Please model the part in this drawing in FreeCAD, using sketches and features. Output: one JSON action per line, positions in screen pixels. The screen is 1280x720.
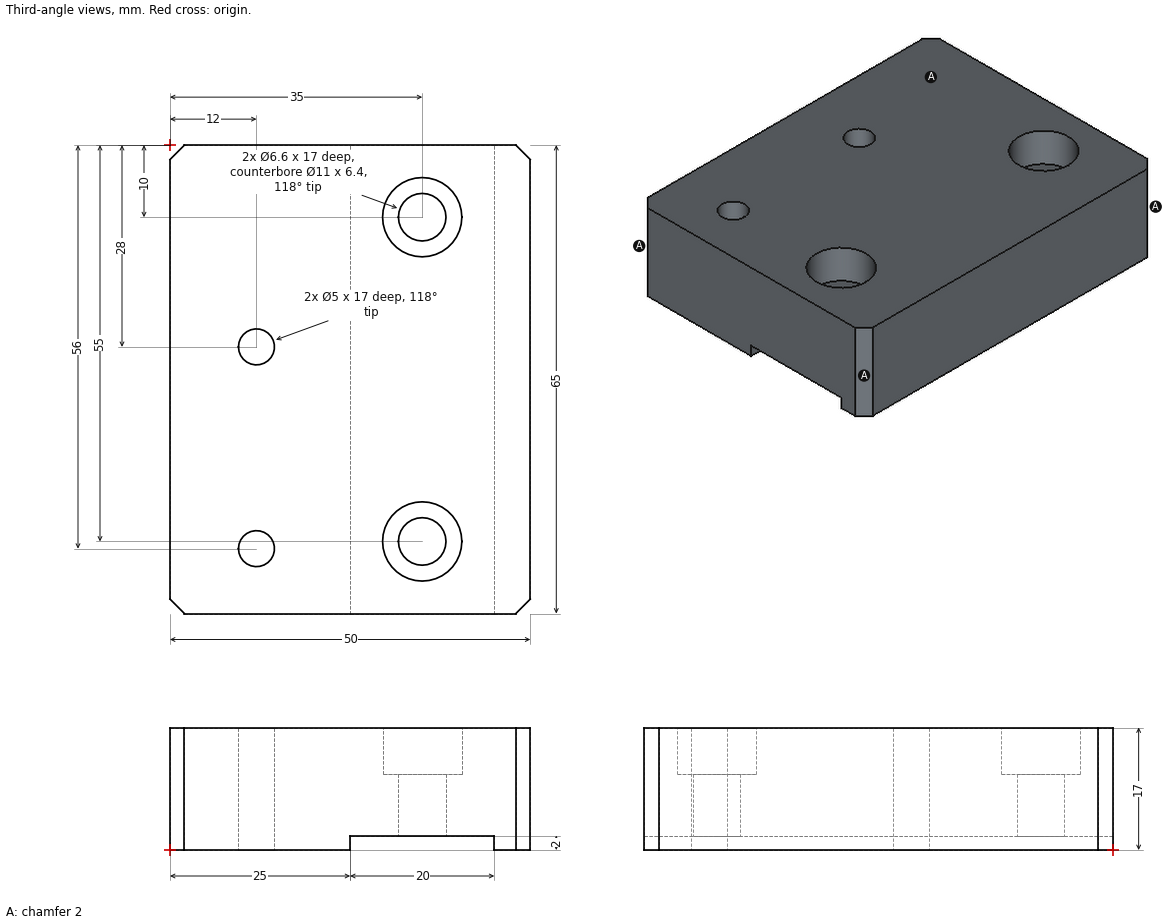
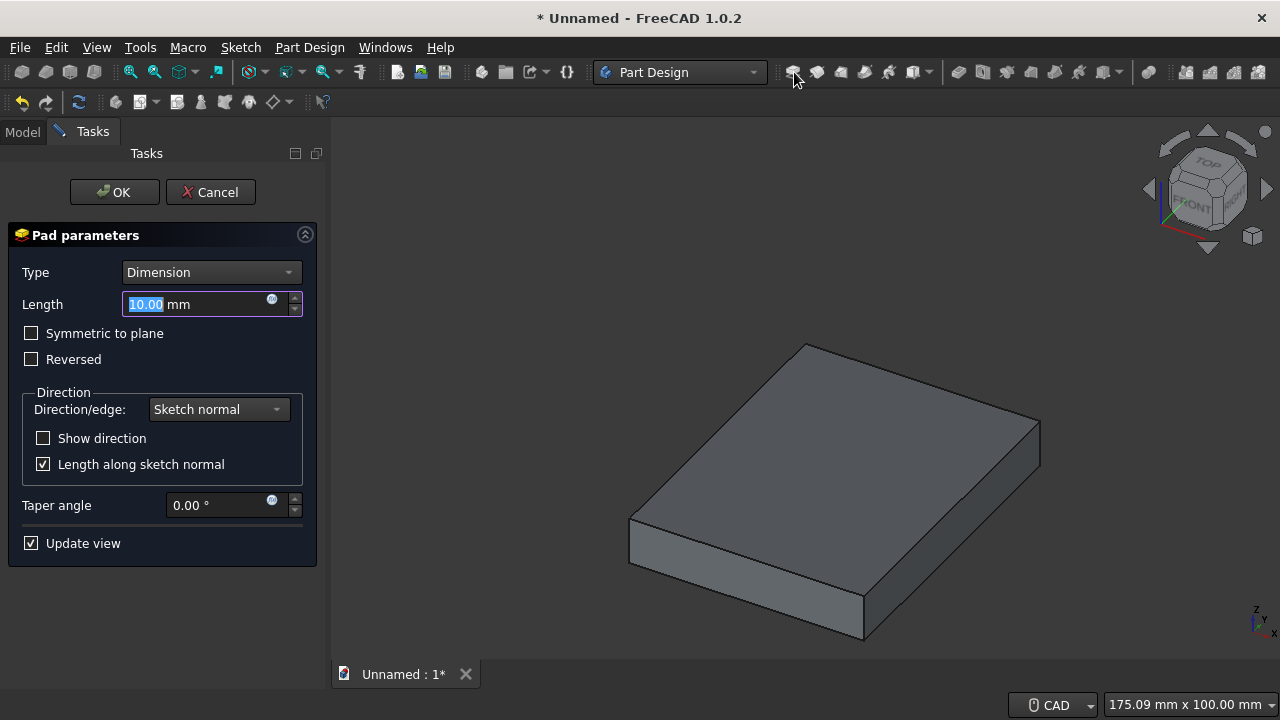
{"action": "type", "text": "17"}
{"action": "key", "text": "Tab"}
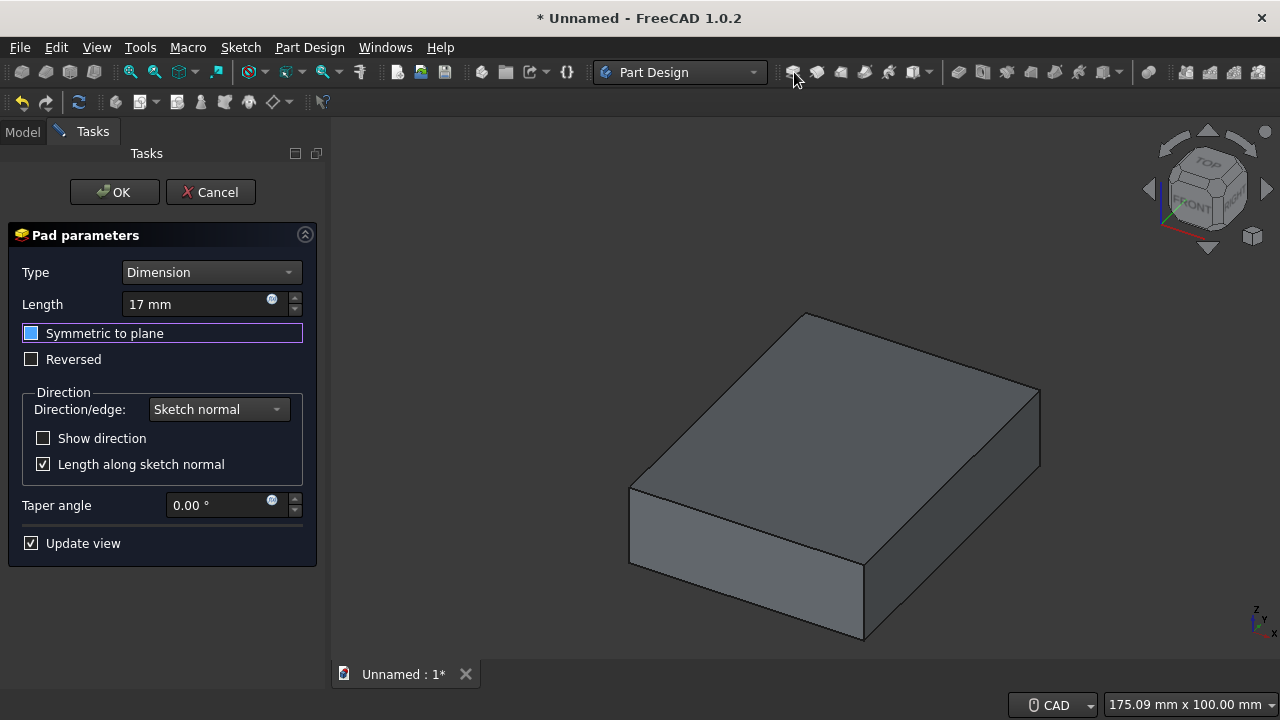
{"action": "left_click", "coordinate": [115, 192]}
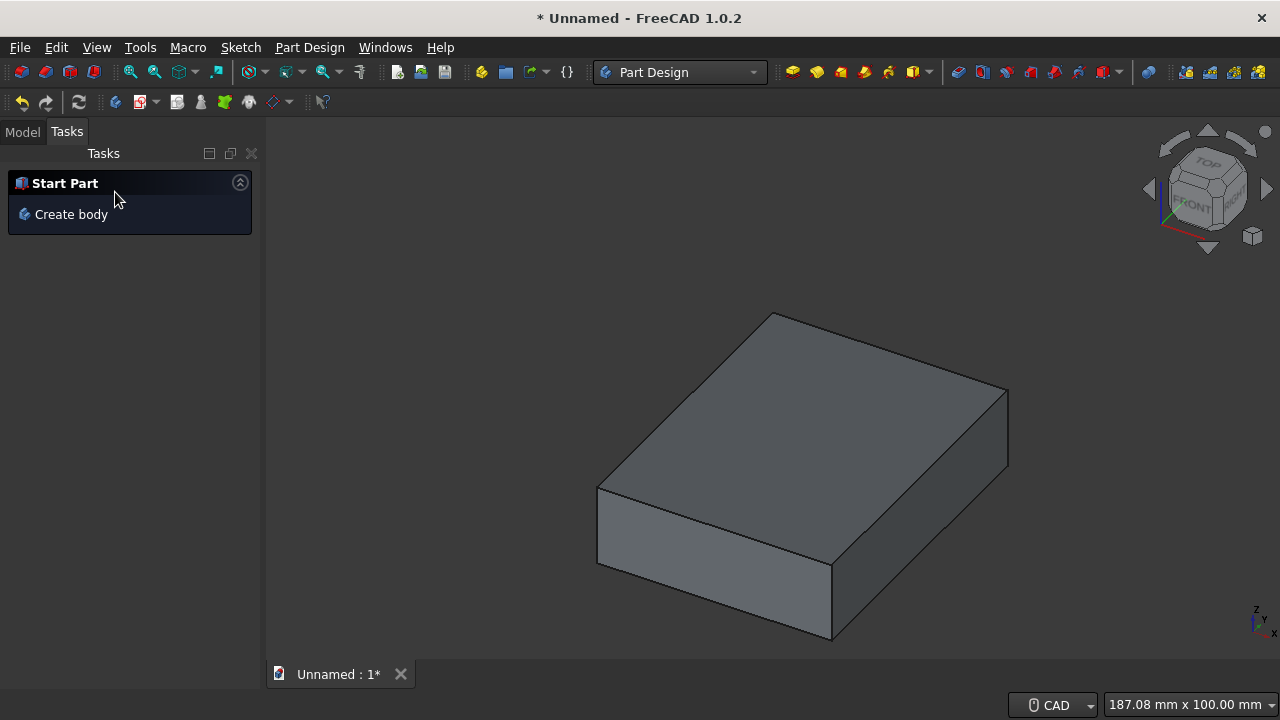
{"action": "left_click", "coordinate": [781, 585]}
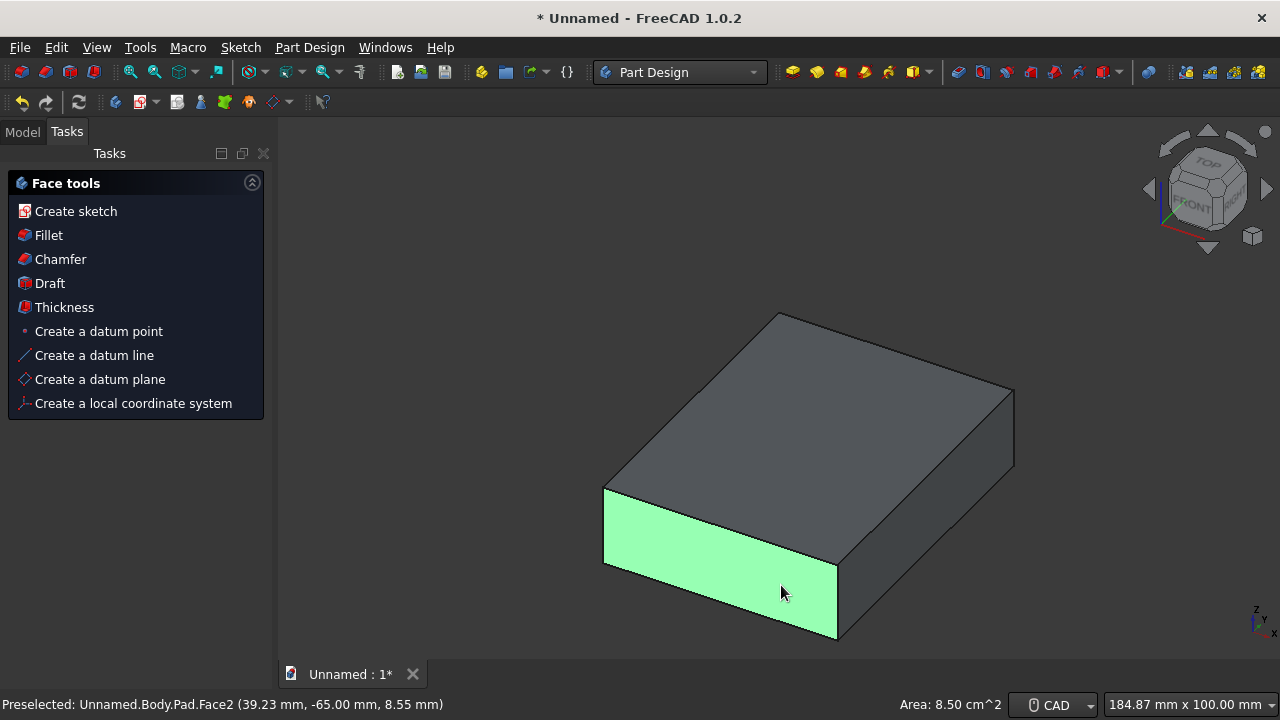
{"action": "left_click", "coordinate": [140, 102]}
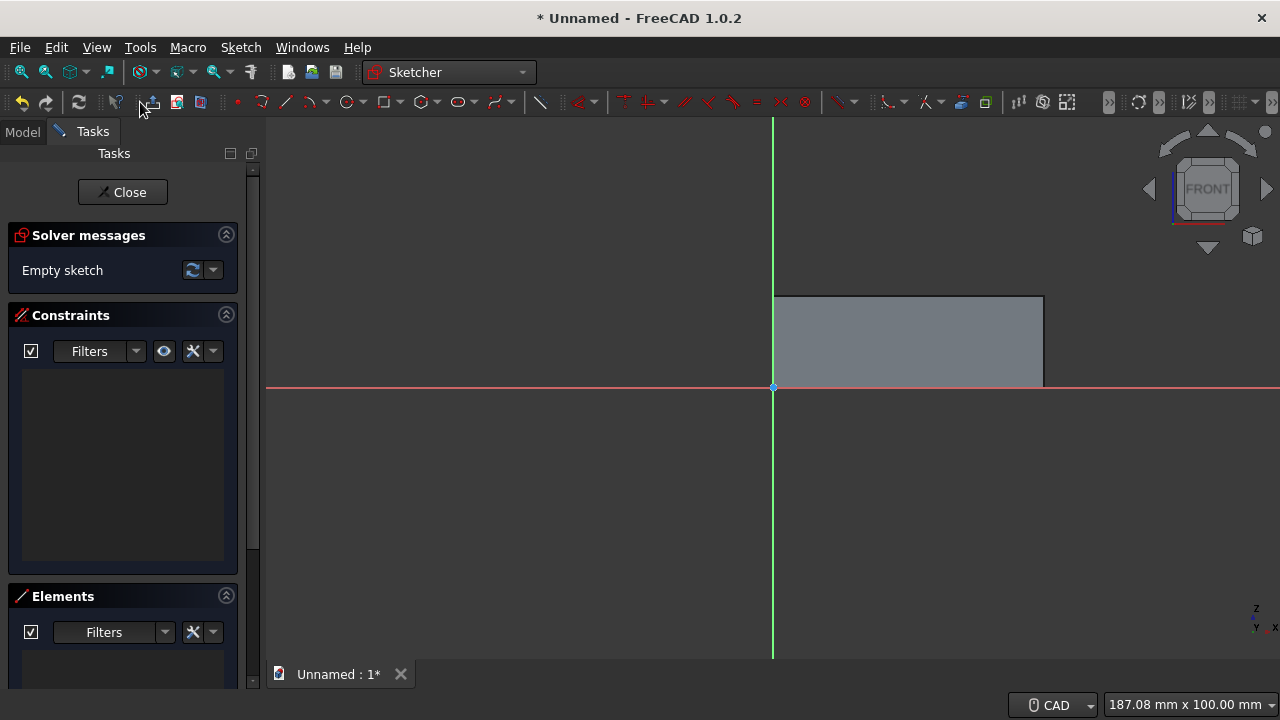
{"action": "scroll", "coordinate": [1050, 378], "scroll_direction": "up", "scroll_amount": 4}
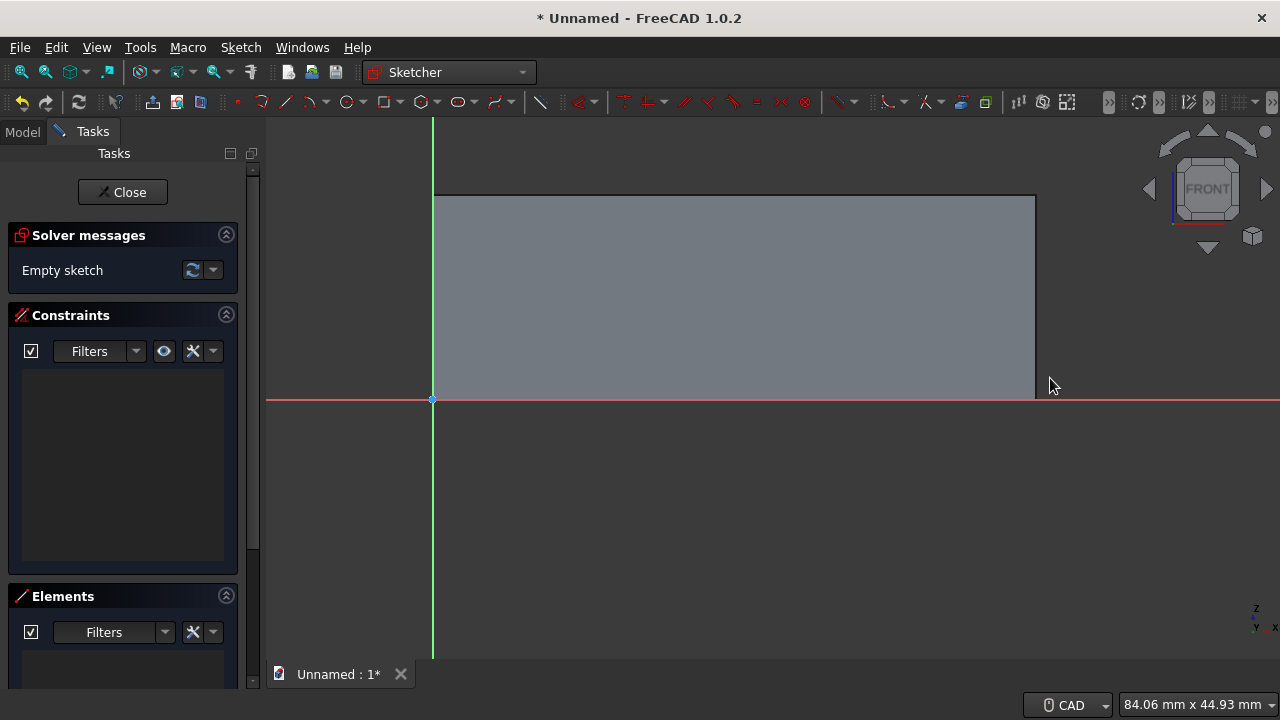
{"action": "left_click", "coordinate": [384, 102]}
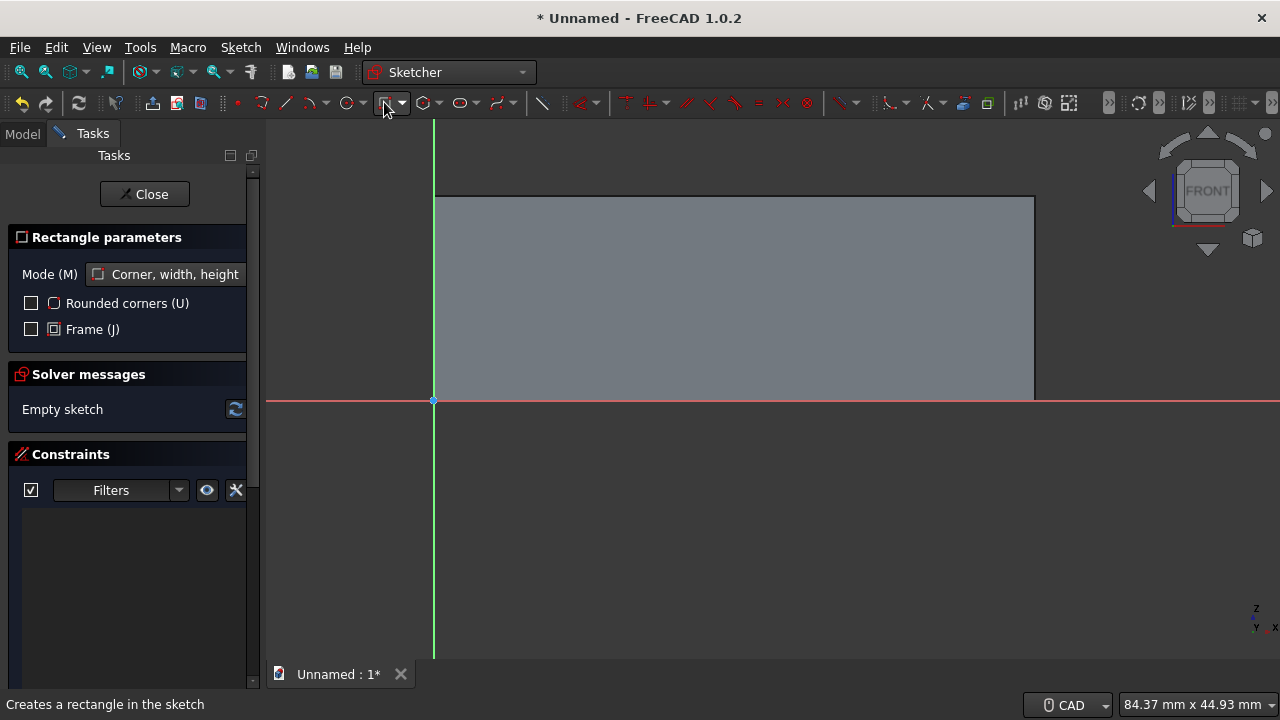
{"action": "left_click", "coordinate": [734, 377]}
{"action": "left_click", "coordinate": [975, 401]}
{"action": "key", "text": "Escape"}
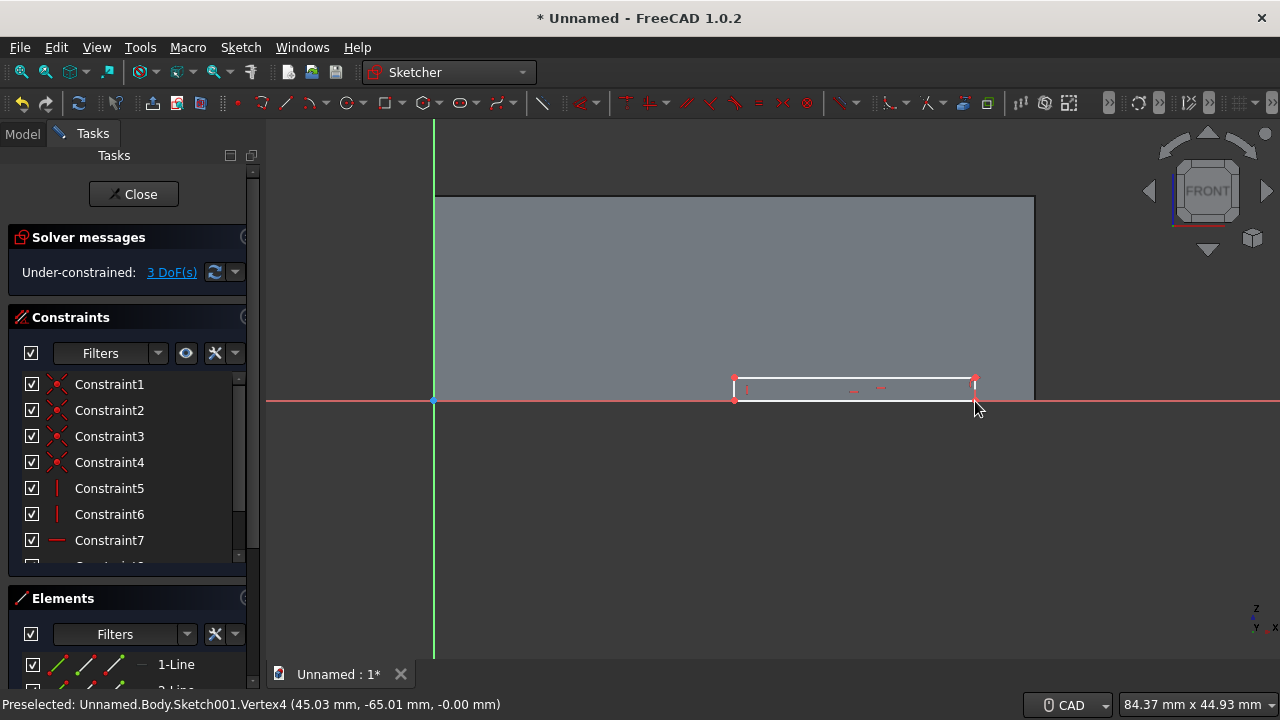
{"action": "scroll", "coordinate": [734, 387], "scroll_direction": "up", "scroll_amount": 3}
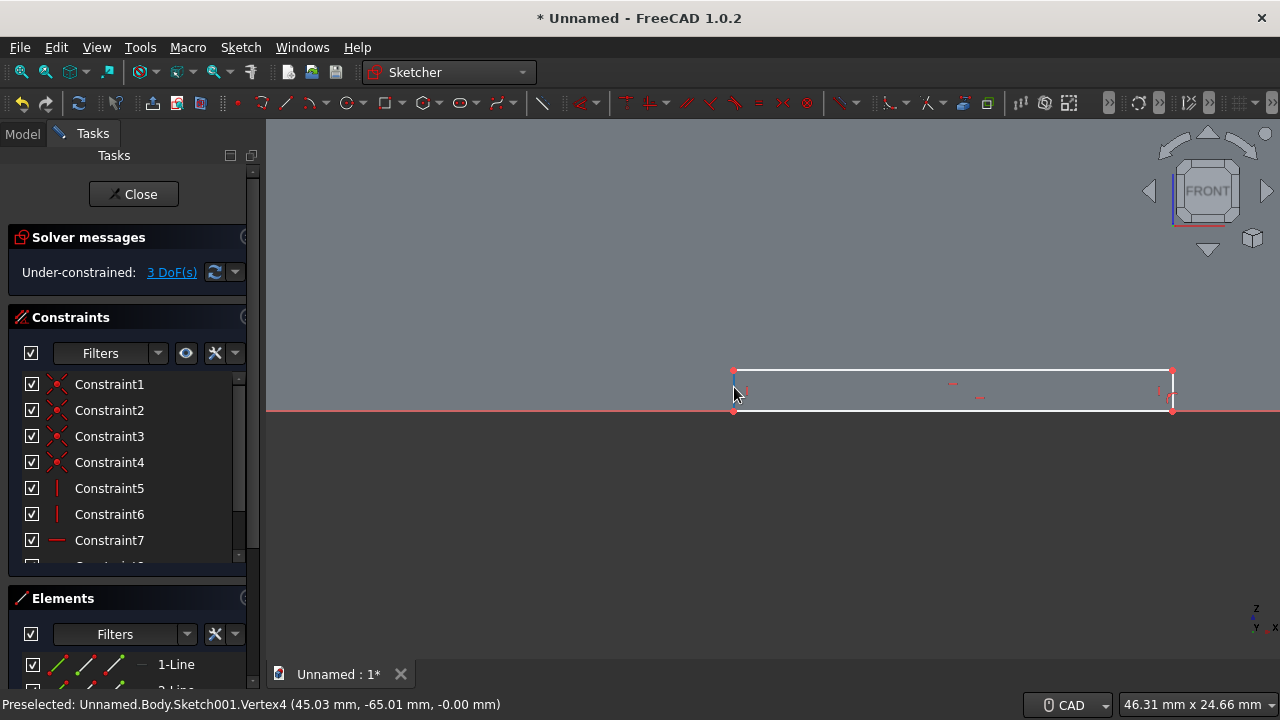
{"action": "left_click", "coordinate": [734, 387]}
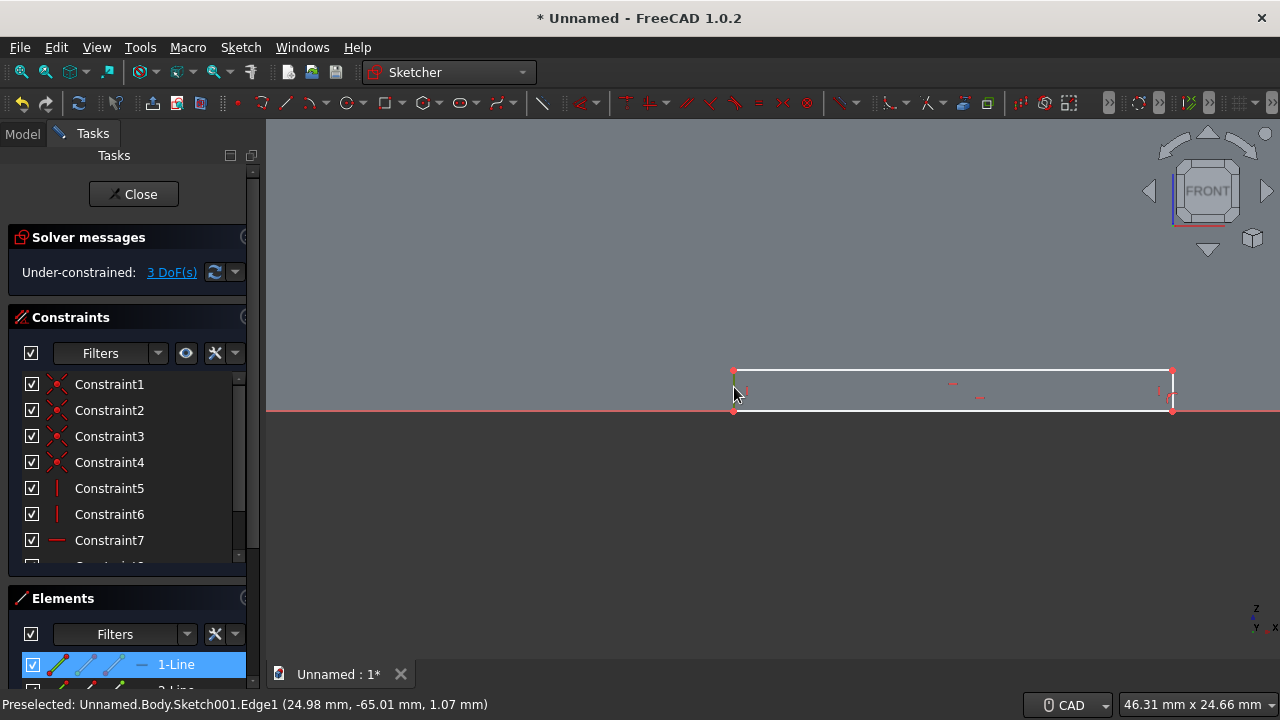
{"action": "key", "text": "i"}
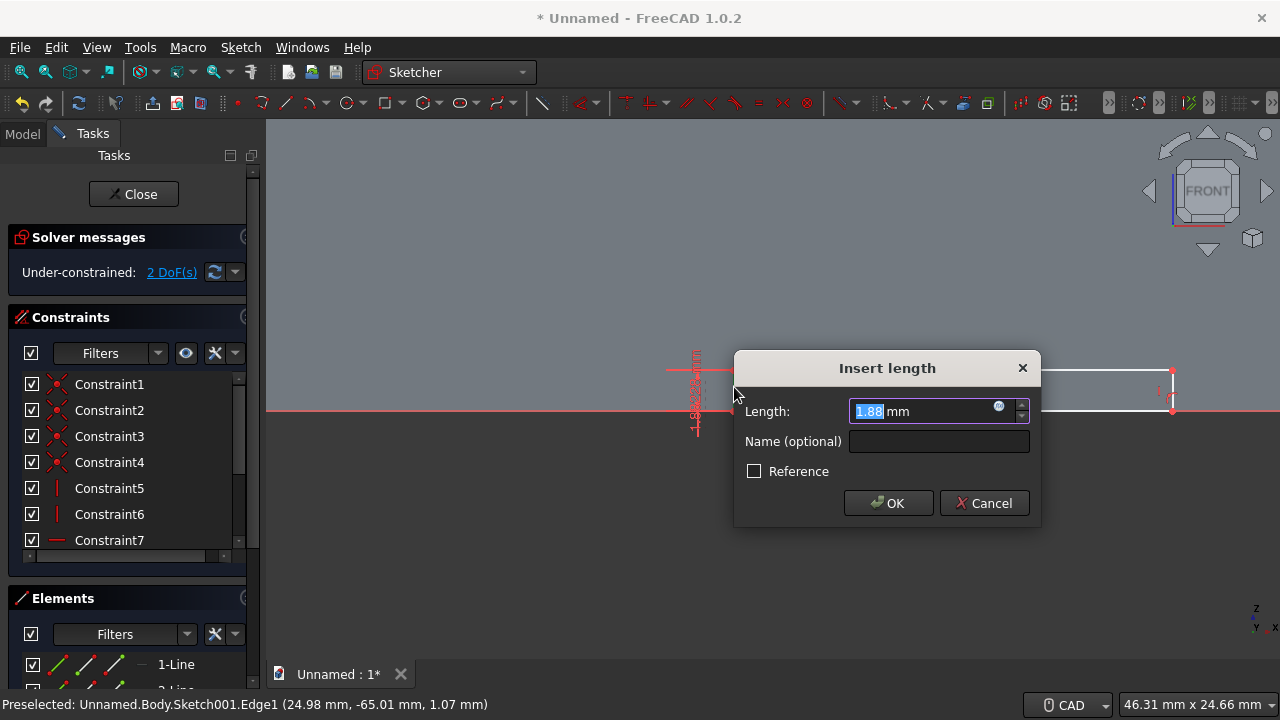
{"action": "type", "text": "2"}
{"action": "key", "text": "Return"}